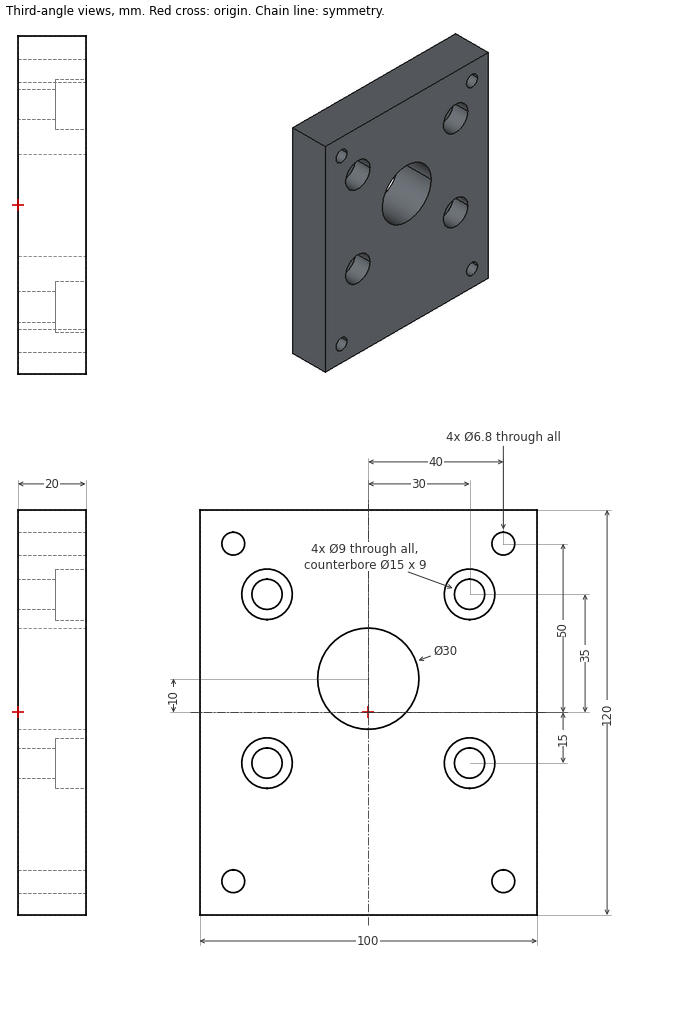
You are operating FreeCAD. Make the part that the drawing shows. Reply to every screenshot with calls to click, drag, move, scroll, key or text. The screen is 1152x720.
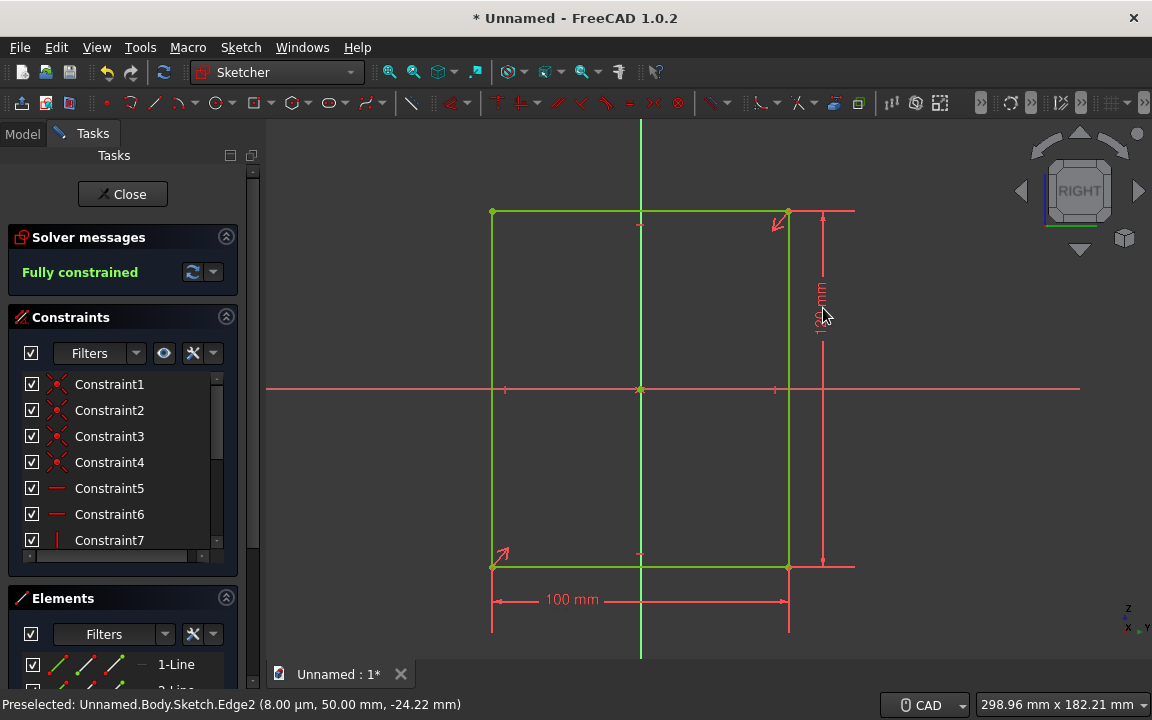
click(123, 194)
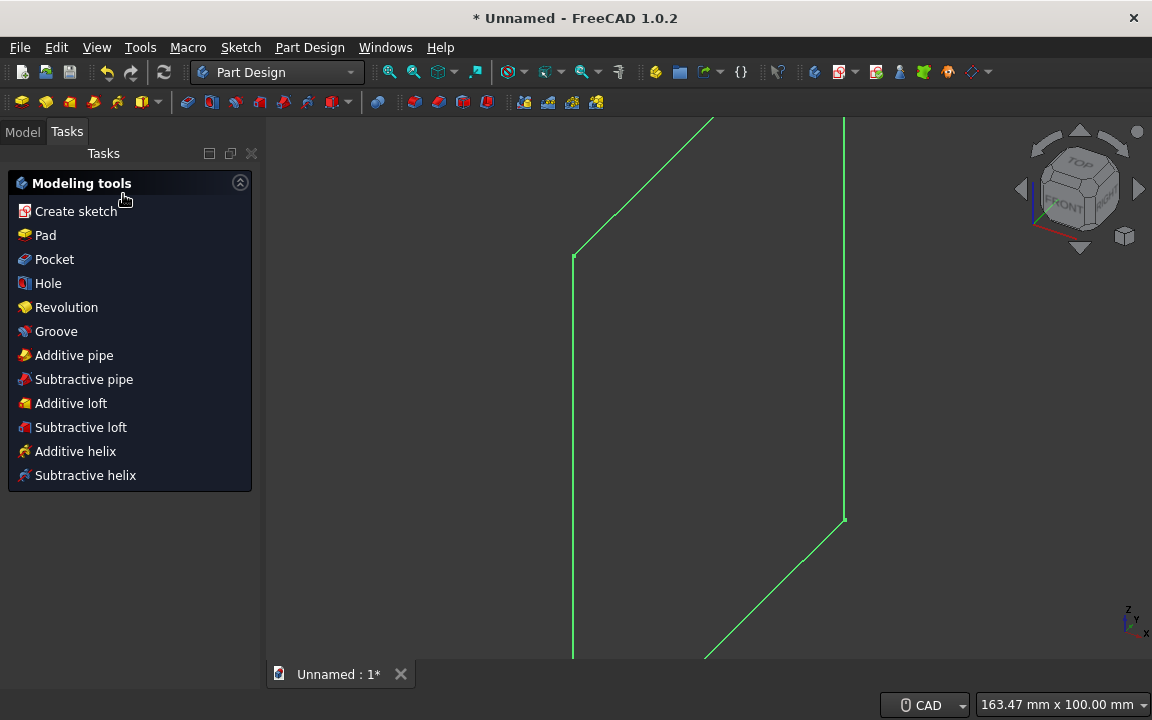
click(22, 102)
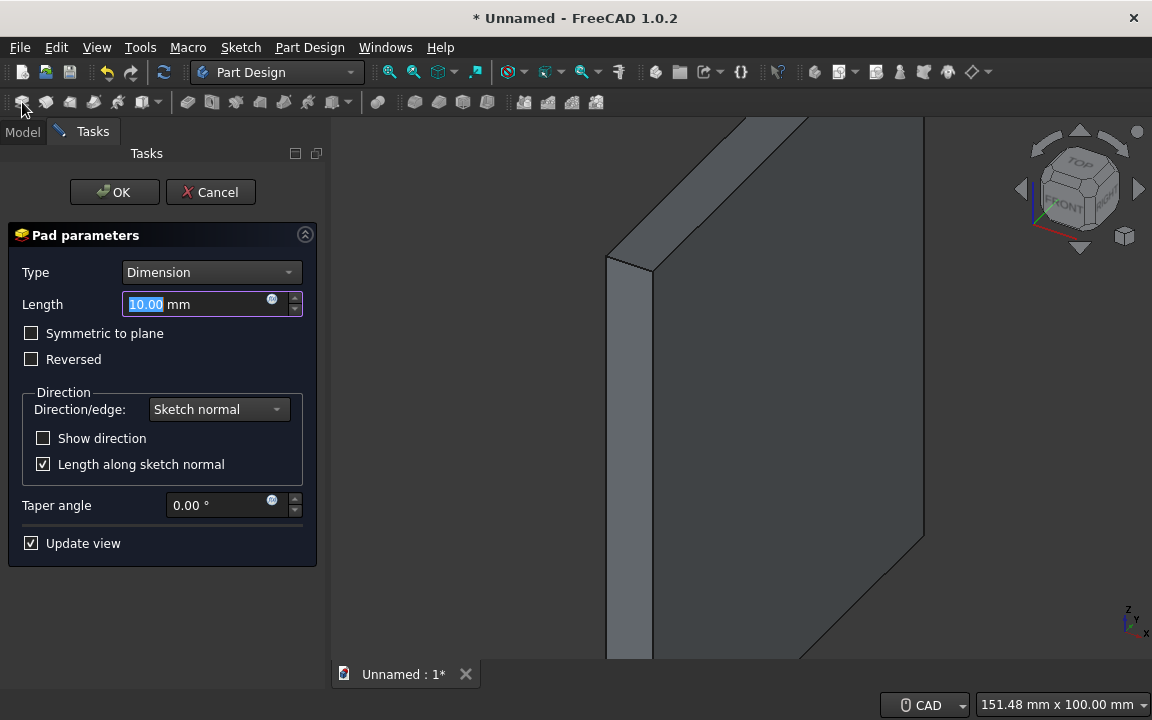
text(20)
key(Tab)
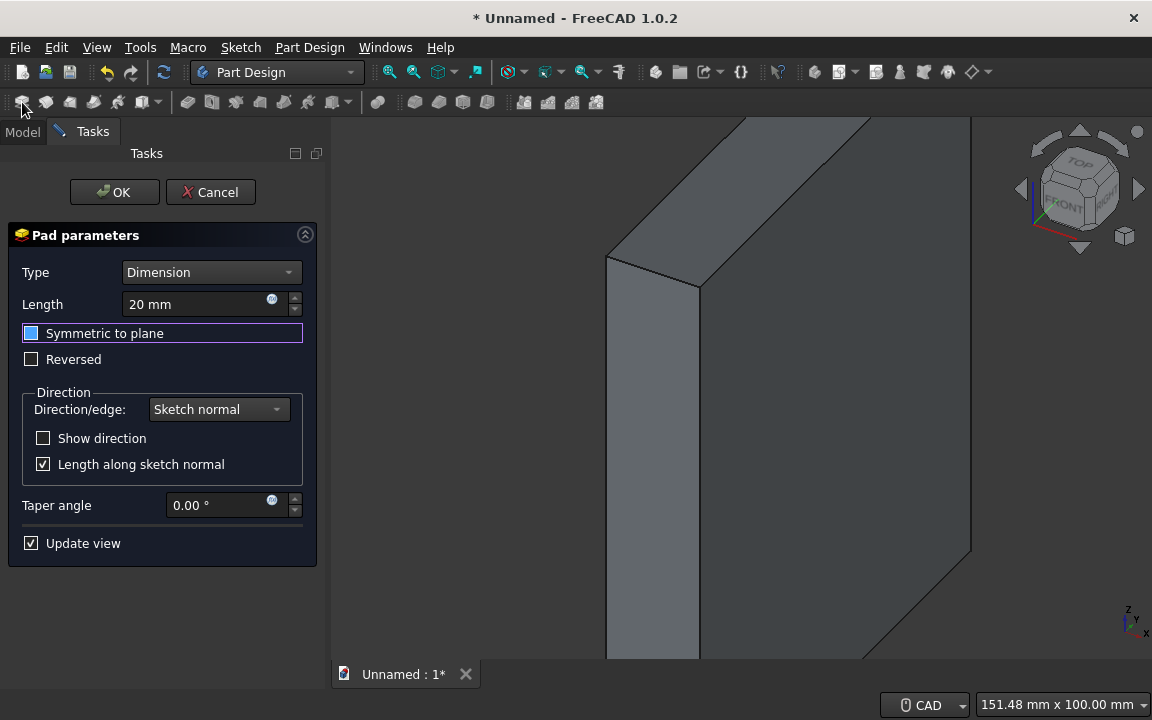
click(115, 192)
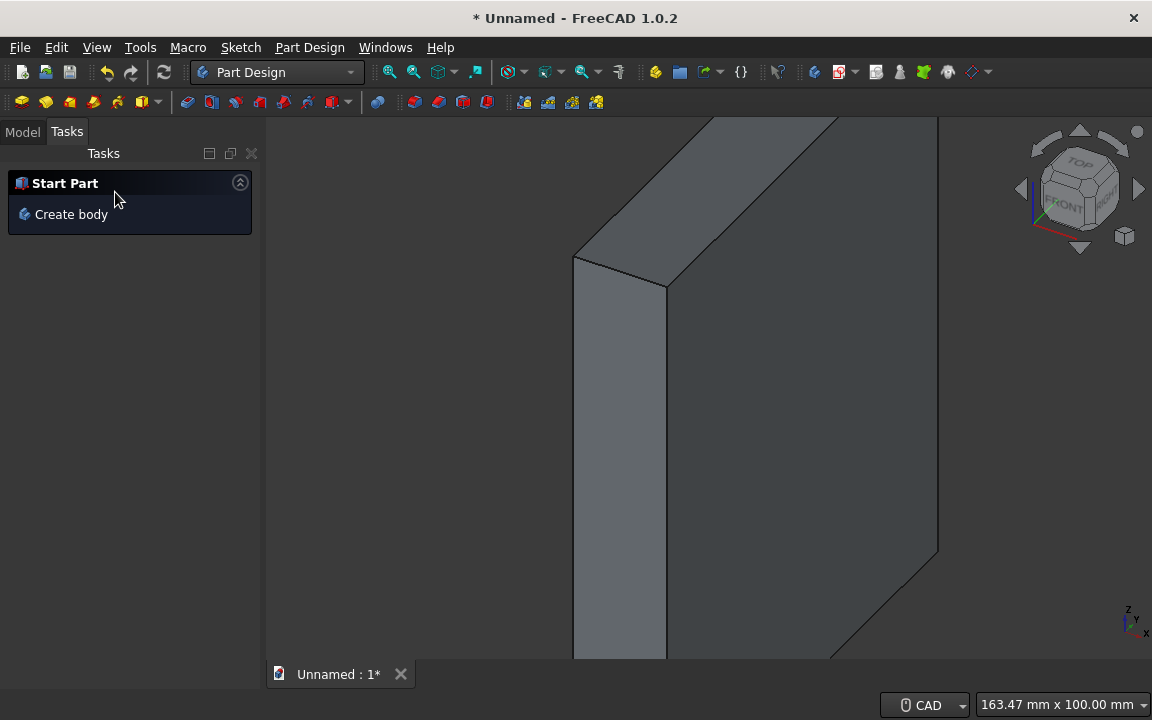
click(390, 72)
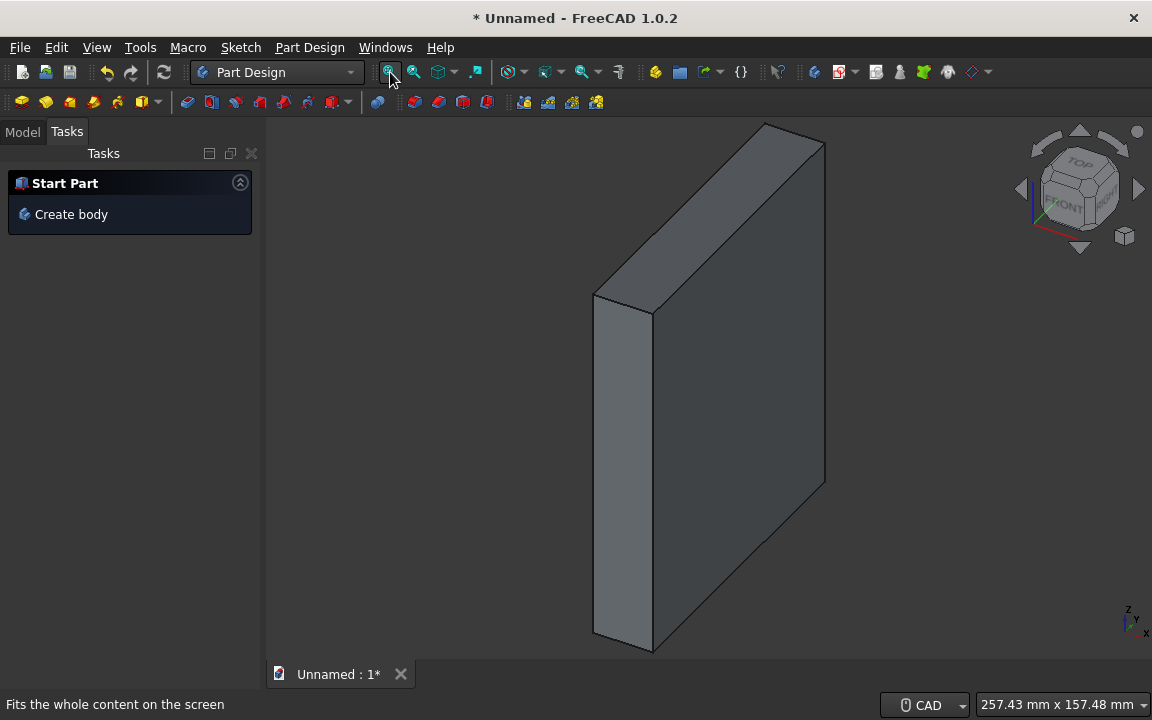
click(739, 397)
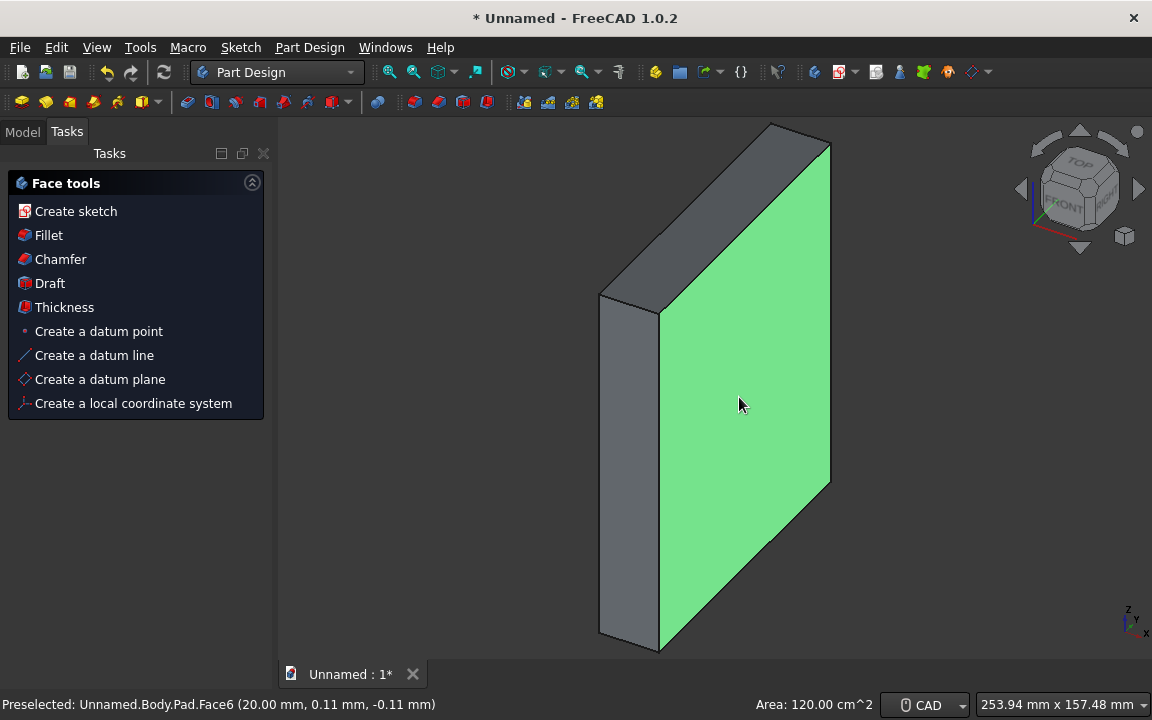
click(840, 72)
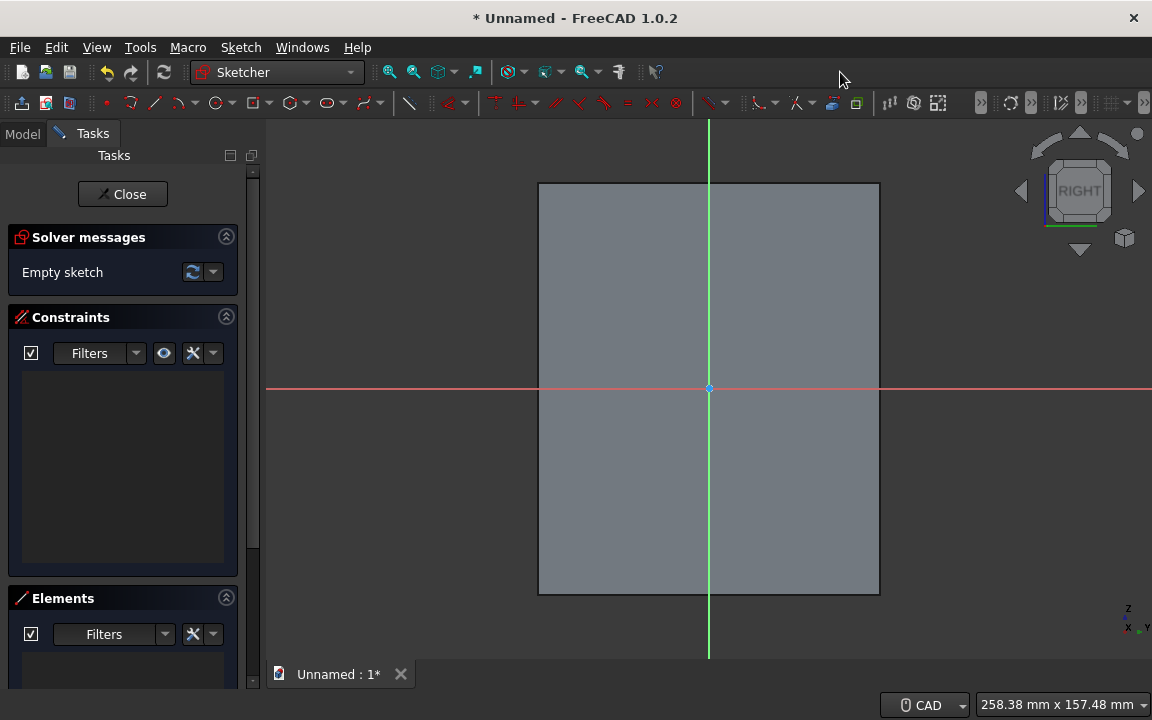
scroll(792, 313, up, 3)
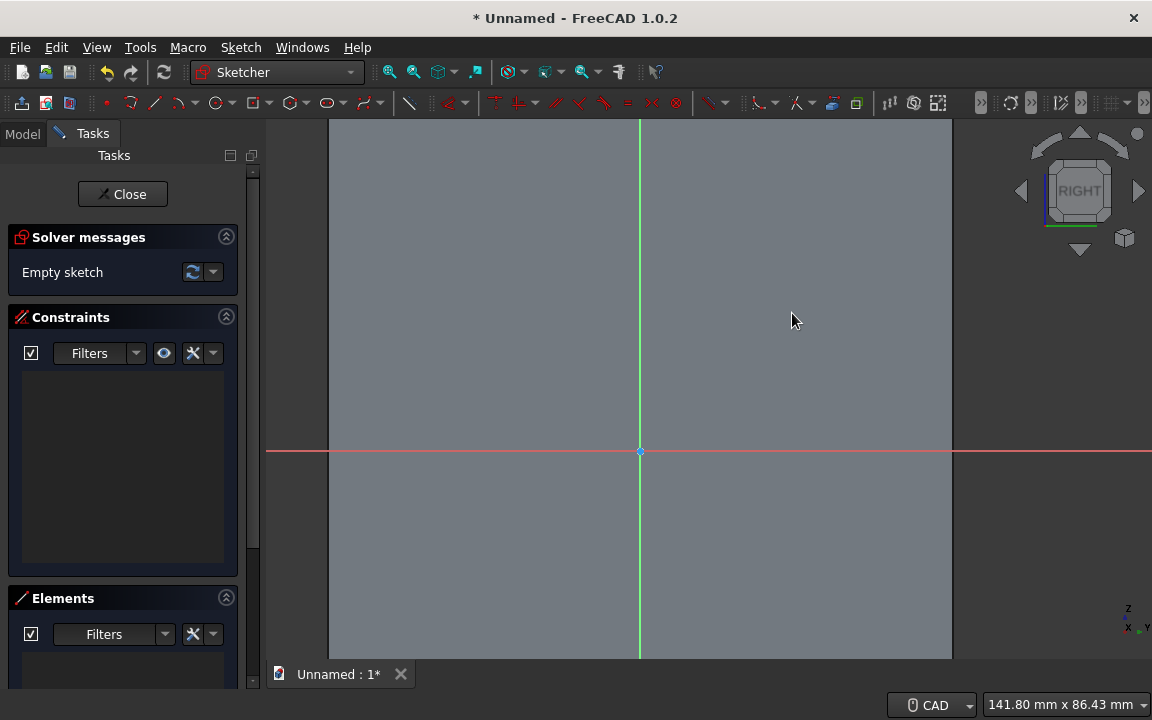
click(216, 104)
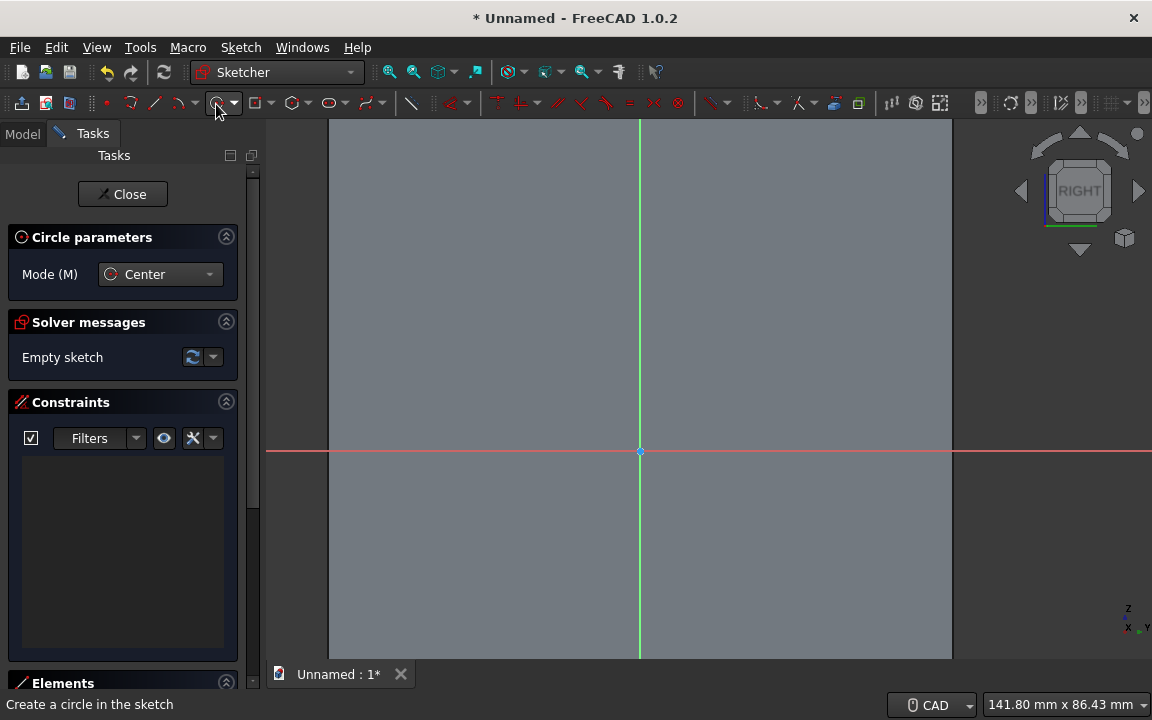
click(828, 233)
click(848, 213)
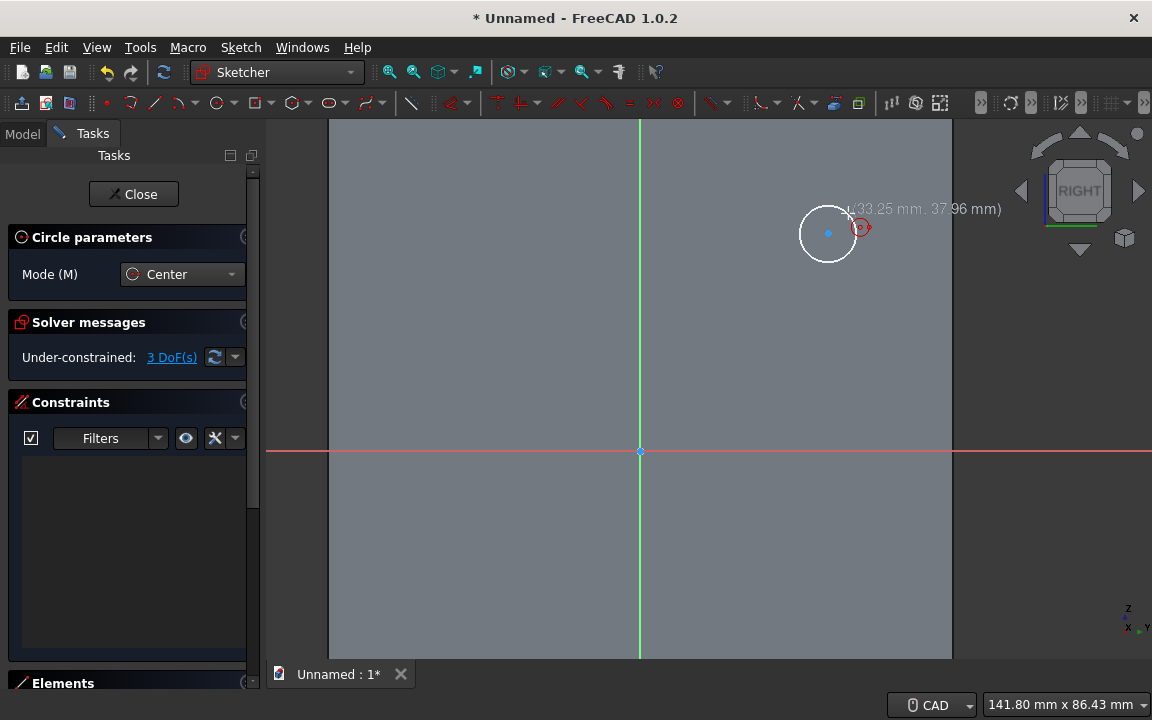
click(828, 545)
click(848, 525)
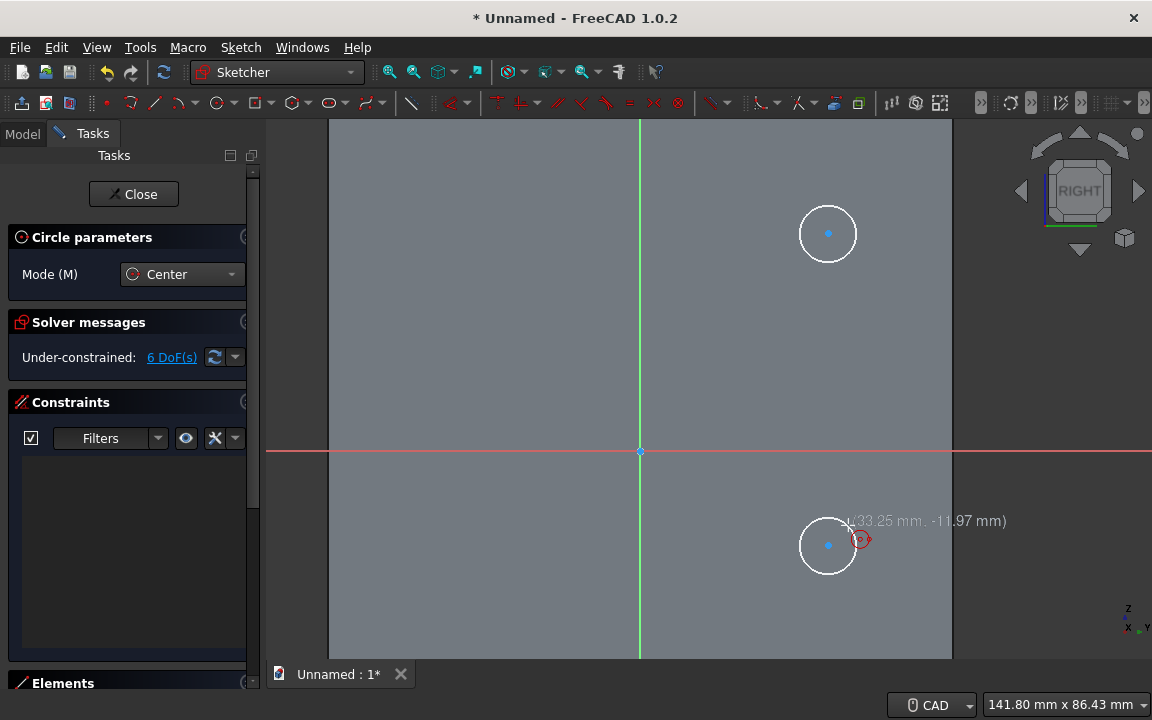
click(453, 233)
click(473, 213)